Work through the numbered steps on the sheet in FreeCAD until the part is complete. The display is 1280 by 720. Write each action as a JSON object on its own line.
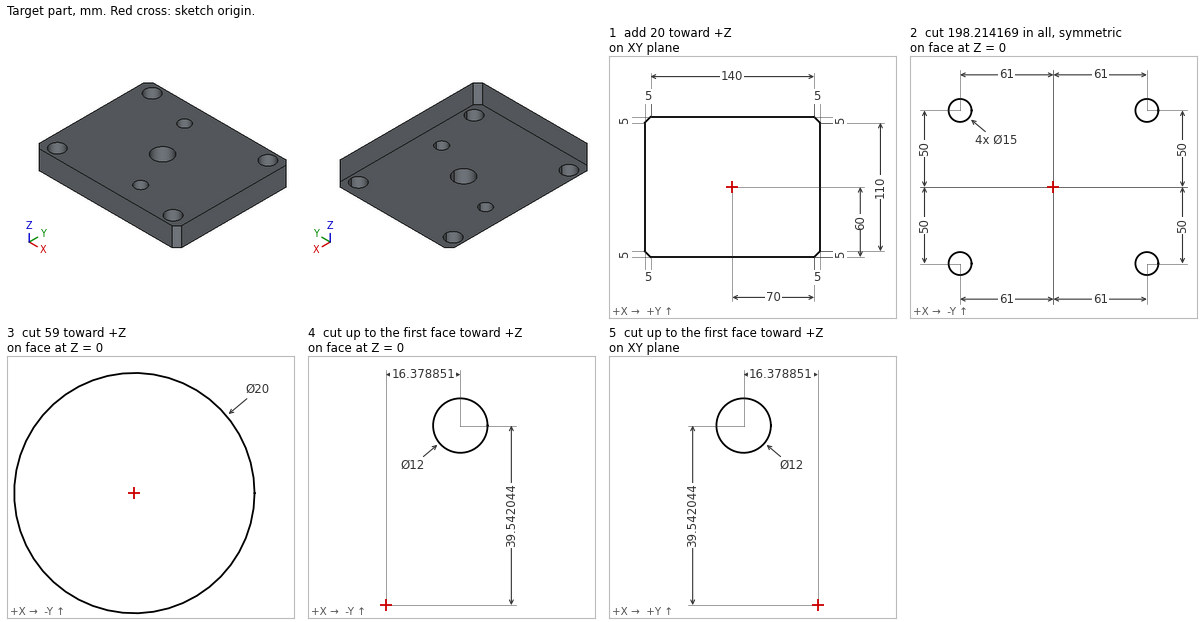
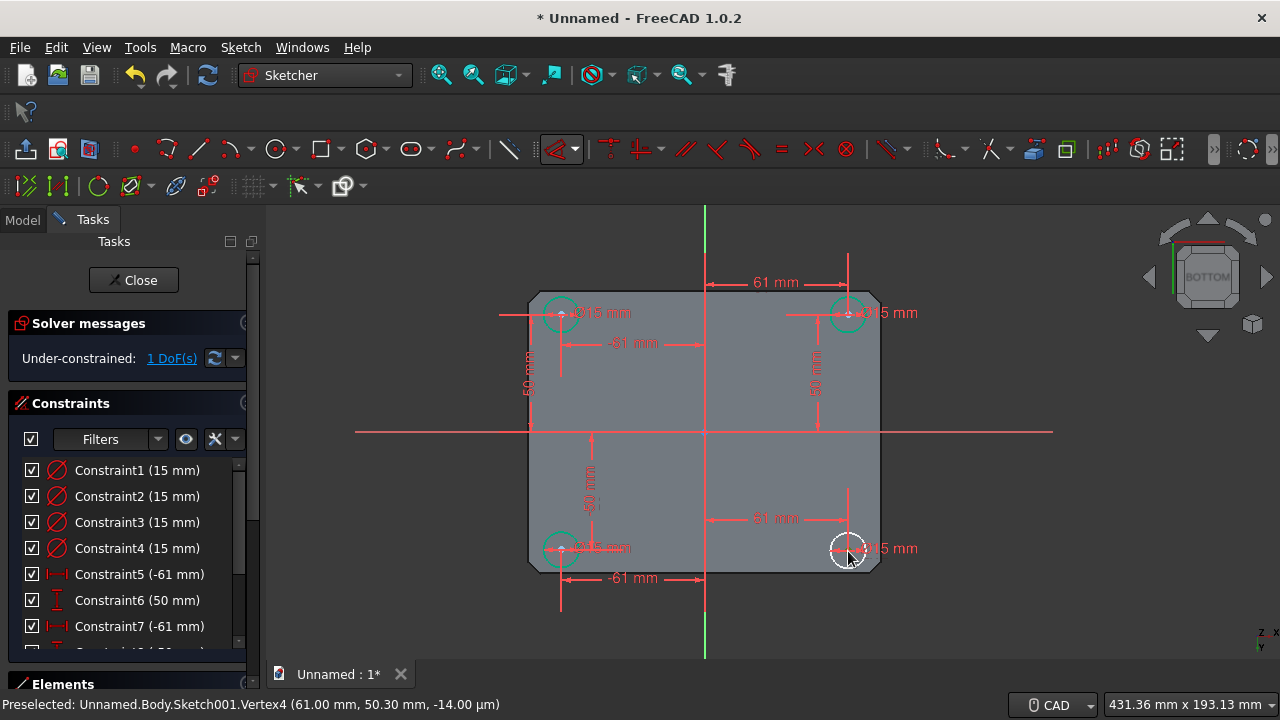
{"action": "key", "text": "i"}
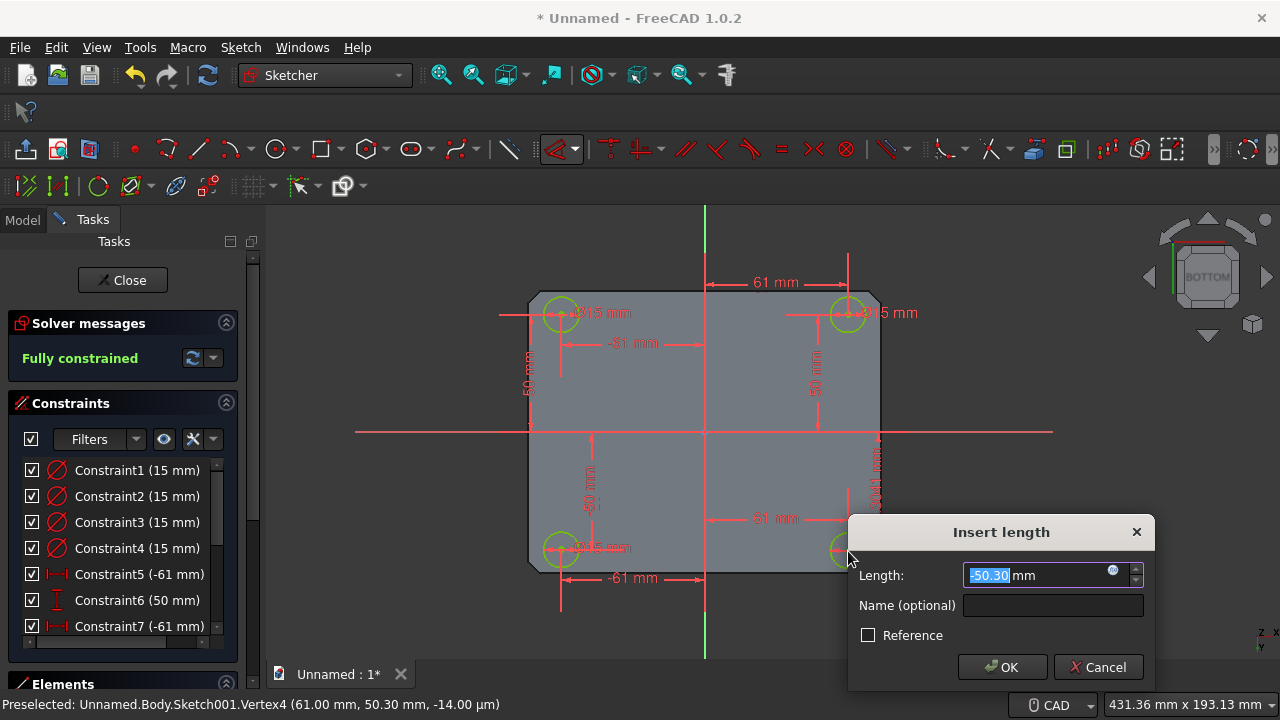
{"action": "type", "text": "-50"}
{"action": "key", "text": "Return"}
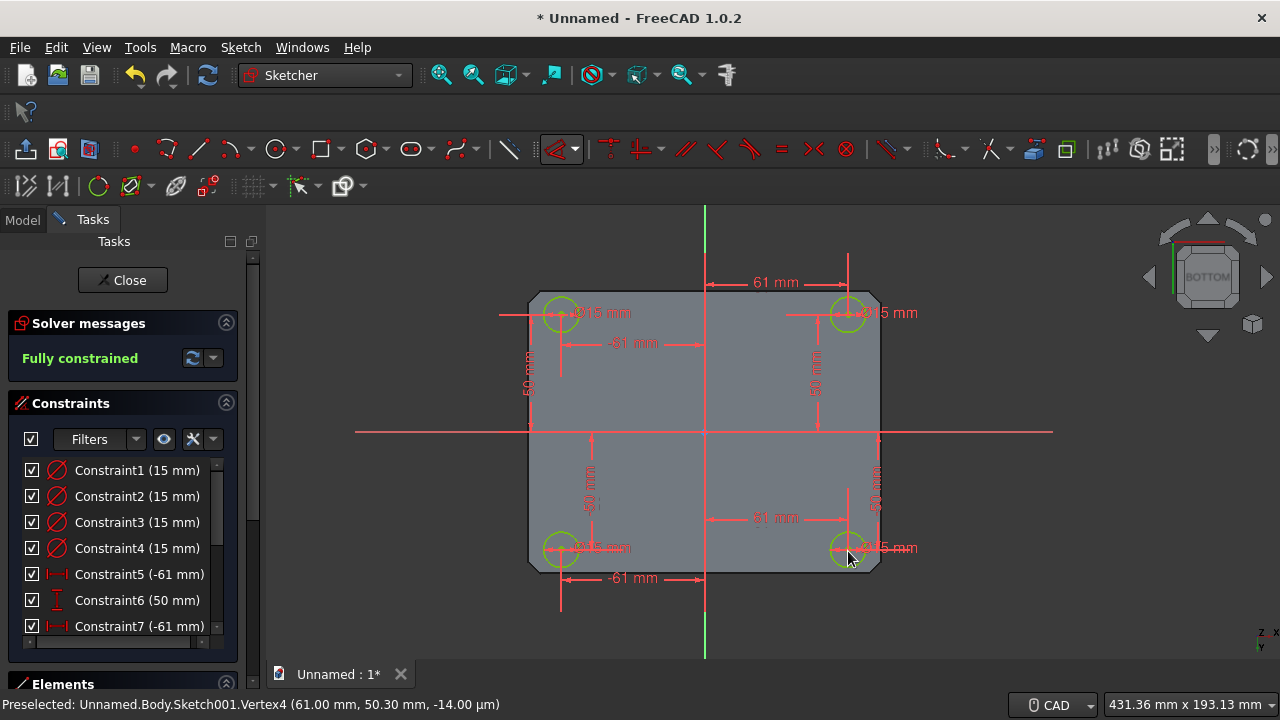
{"action": "left_click", "coordinate": [123, 280]}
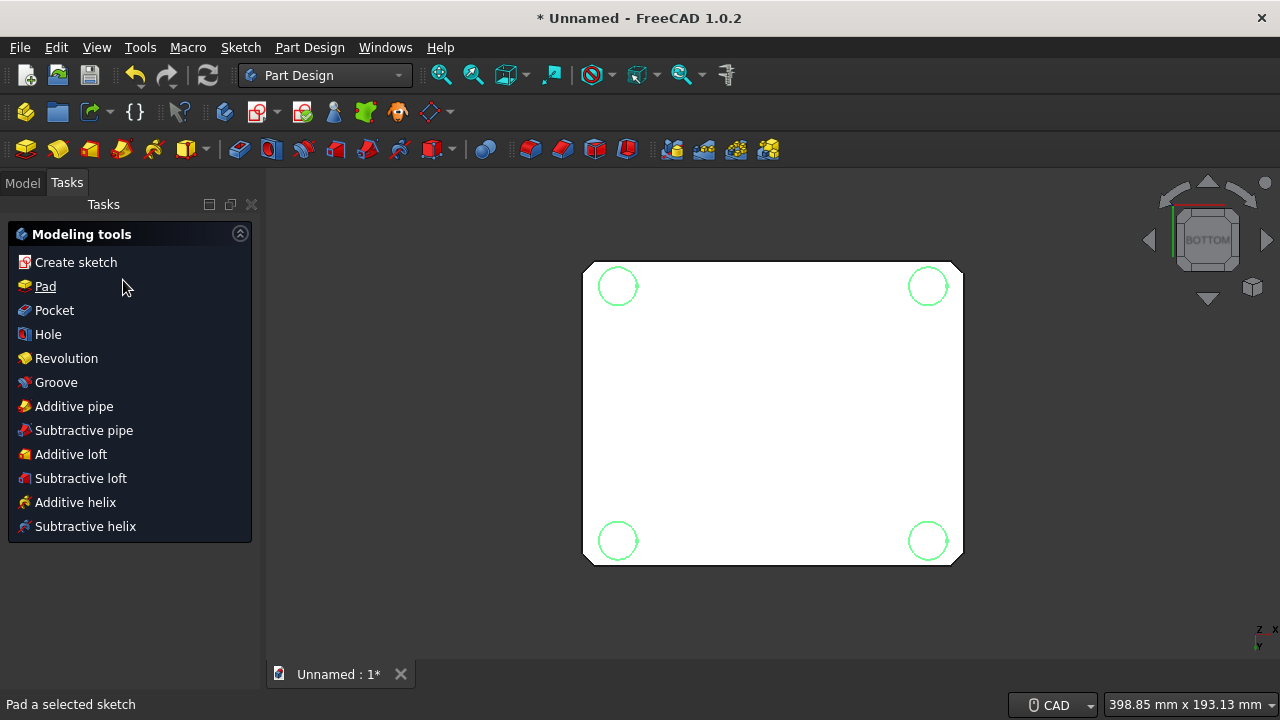
{"action": "left_click", "coordinate": [240, 150]}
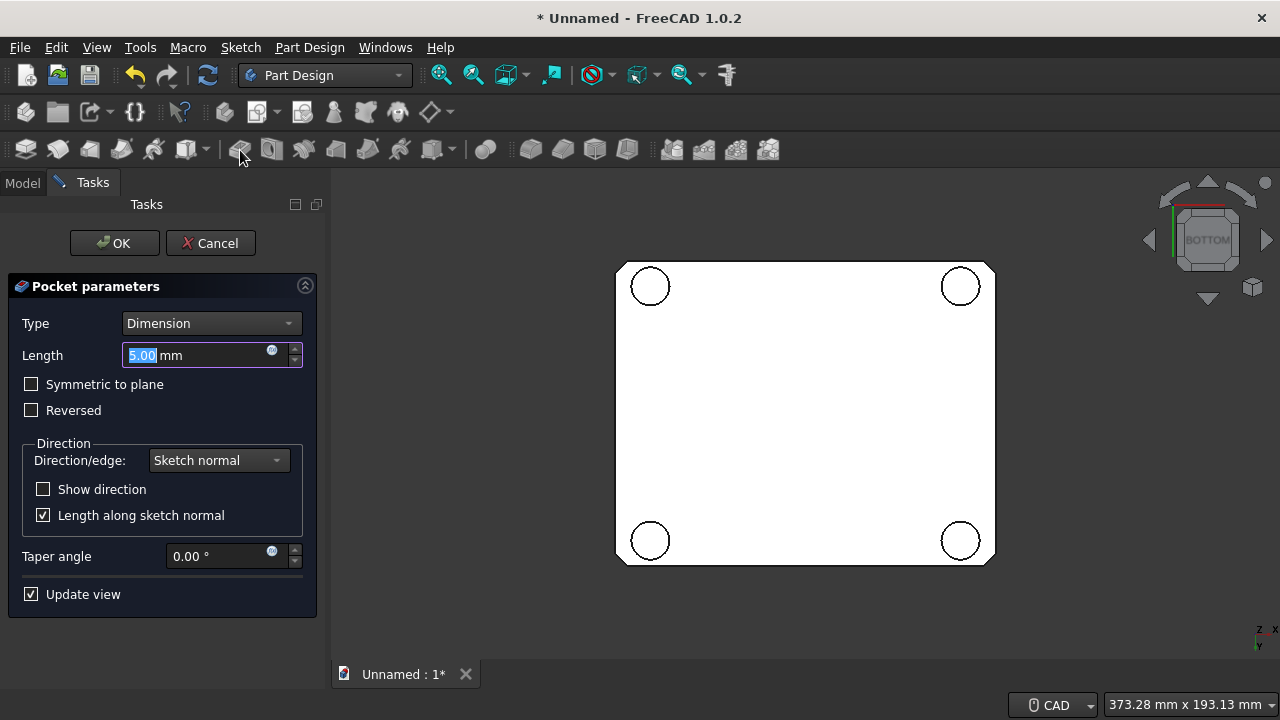
{"action": "type", "text": "198.214169"}
{"action": "key", "text": "Tab"}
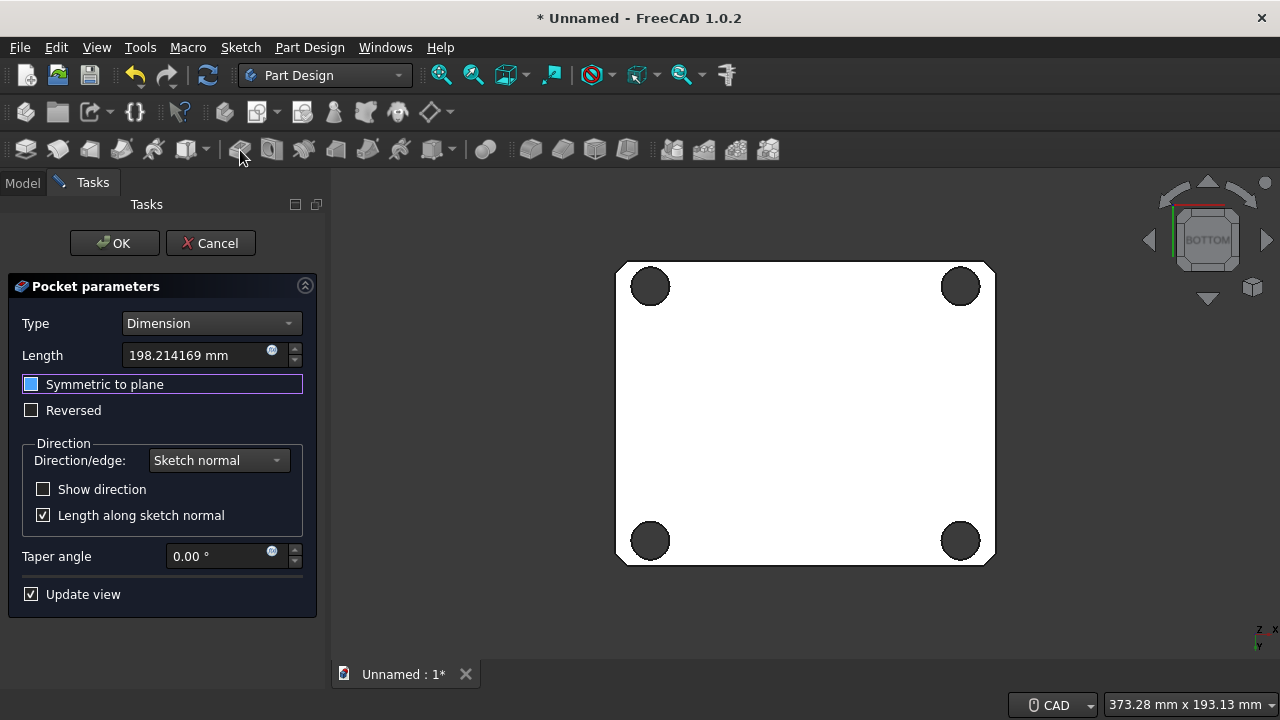
{"action": "left_click", "coordinate": [30, 384]}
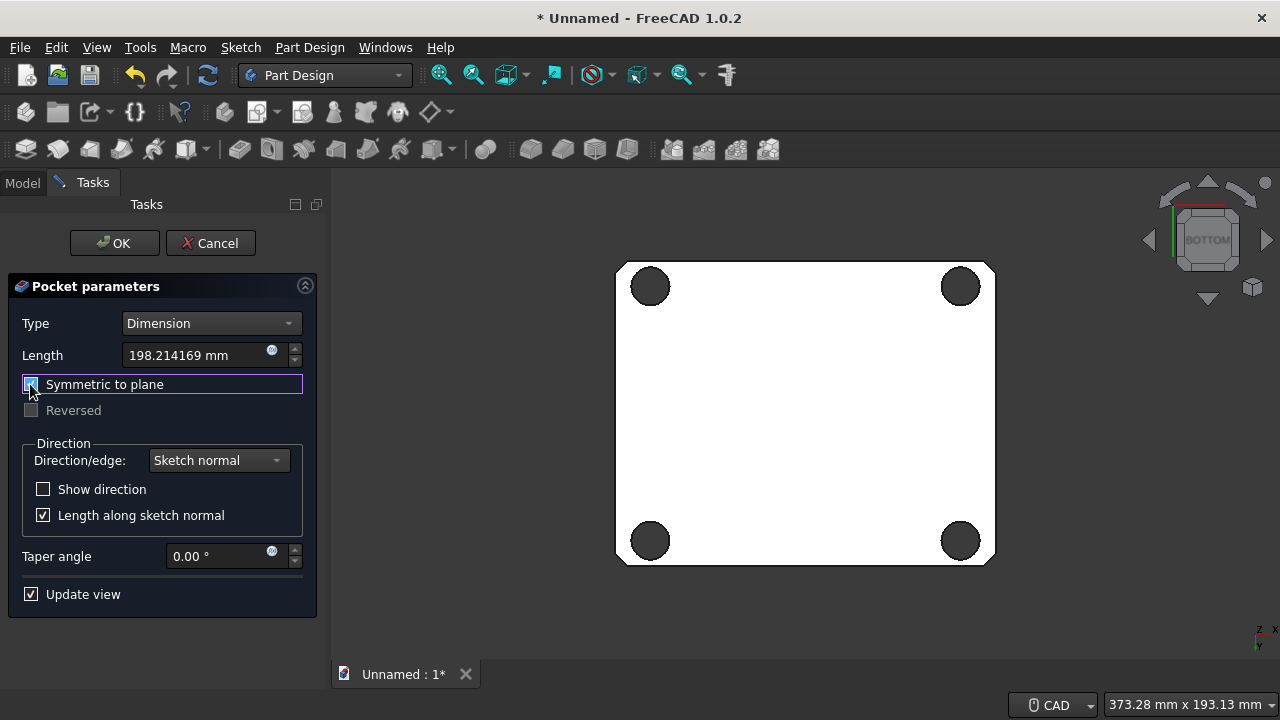
{"action": "left_click", "coordinate": [115, 243]}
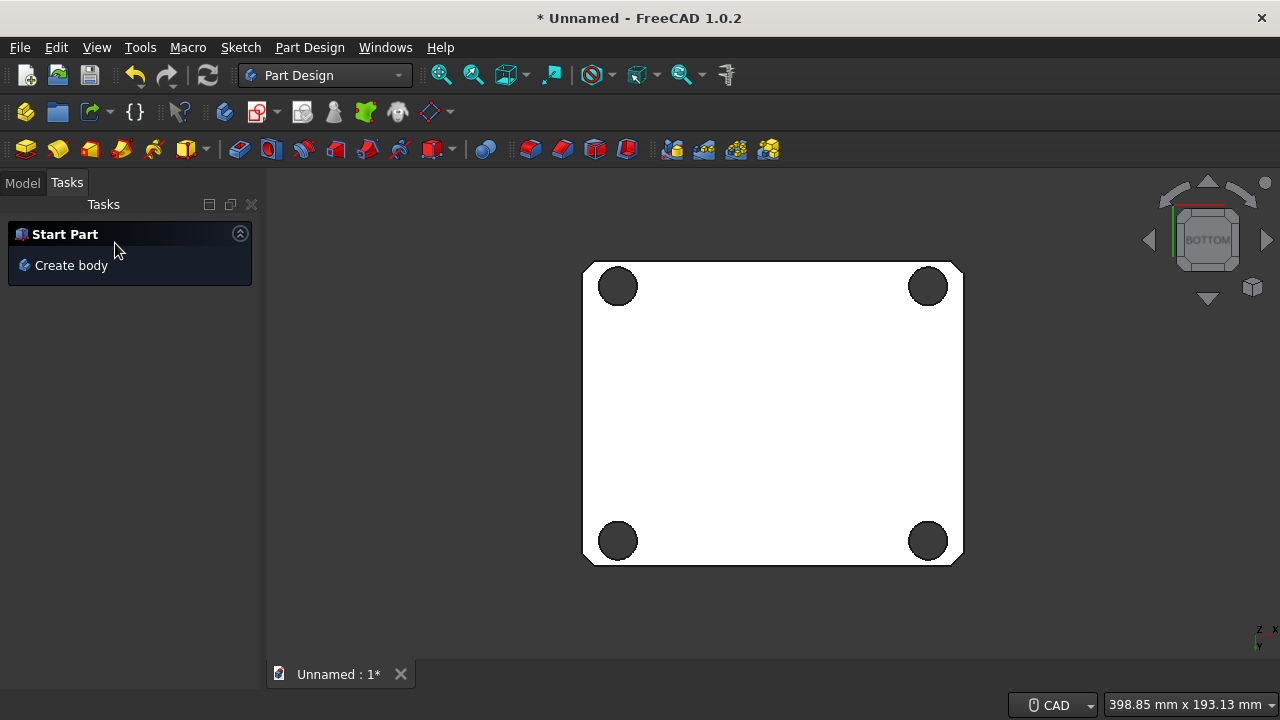
{"action": "left_click", "coordinate": [773, 413]}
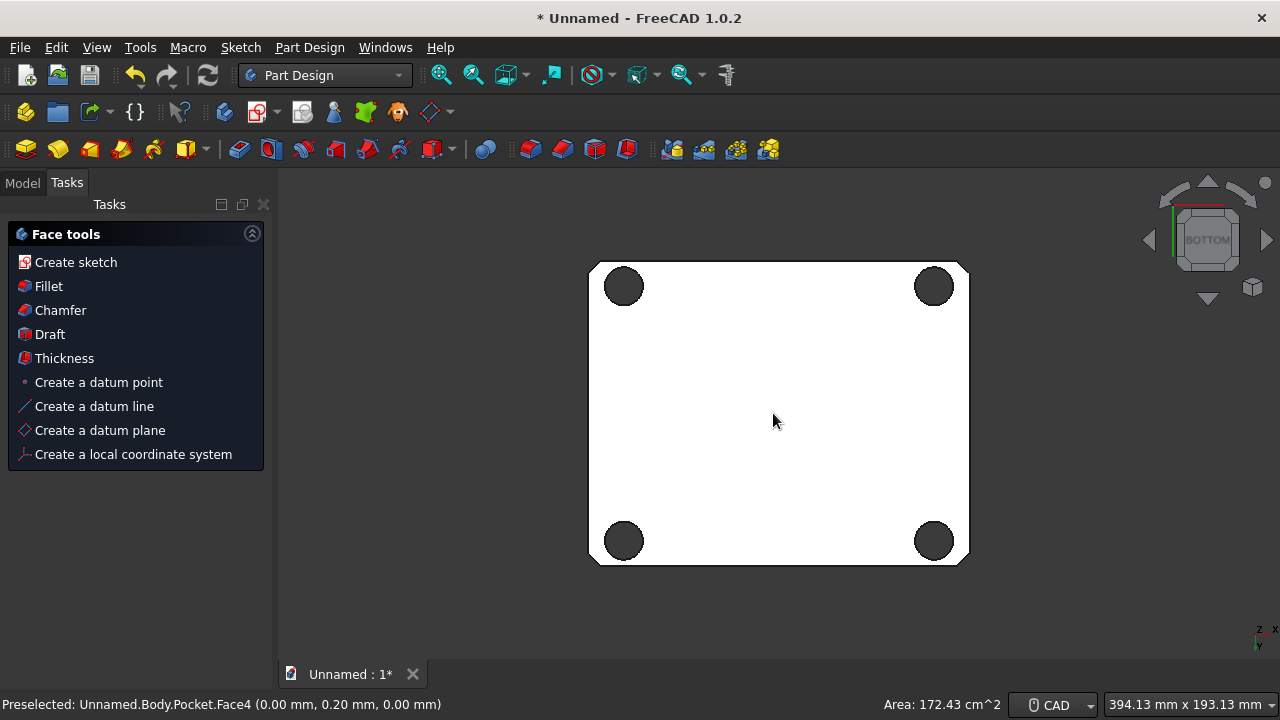
{"action": "left_click", "coordinate": [258, 112]}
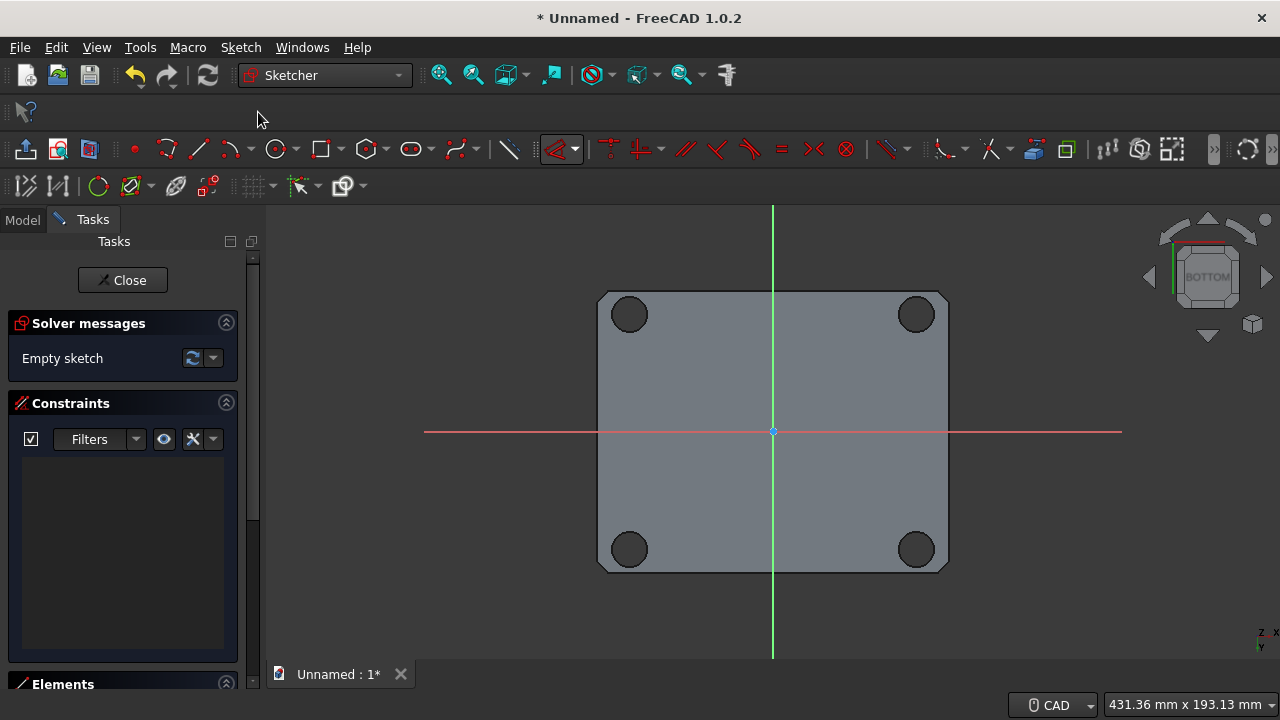
{"action": "scroll", "coordinate": [787, 432], "scroll_direction": "up", "scroll_amount": 9}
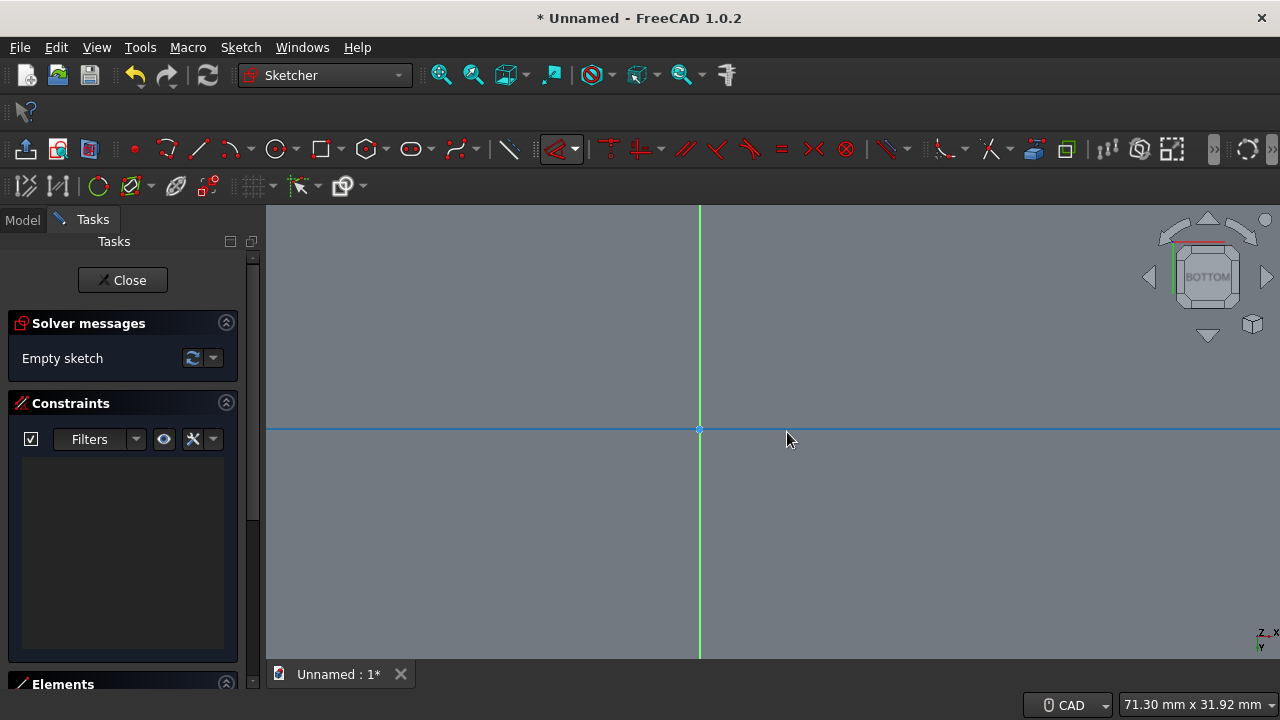
{"action": "left_click", "coordinate": [276, 150]}